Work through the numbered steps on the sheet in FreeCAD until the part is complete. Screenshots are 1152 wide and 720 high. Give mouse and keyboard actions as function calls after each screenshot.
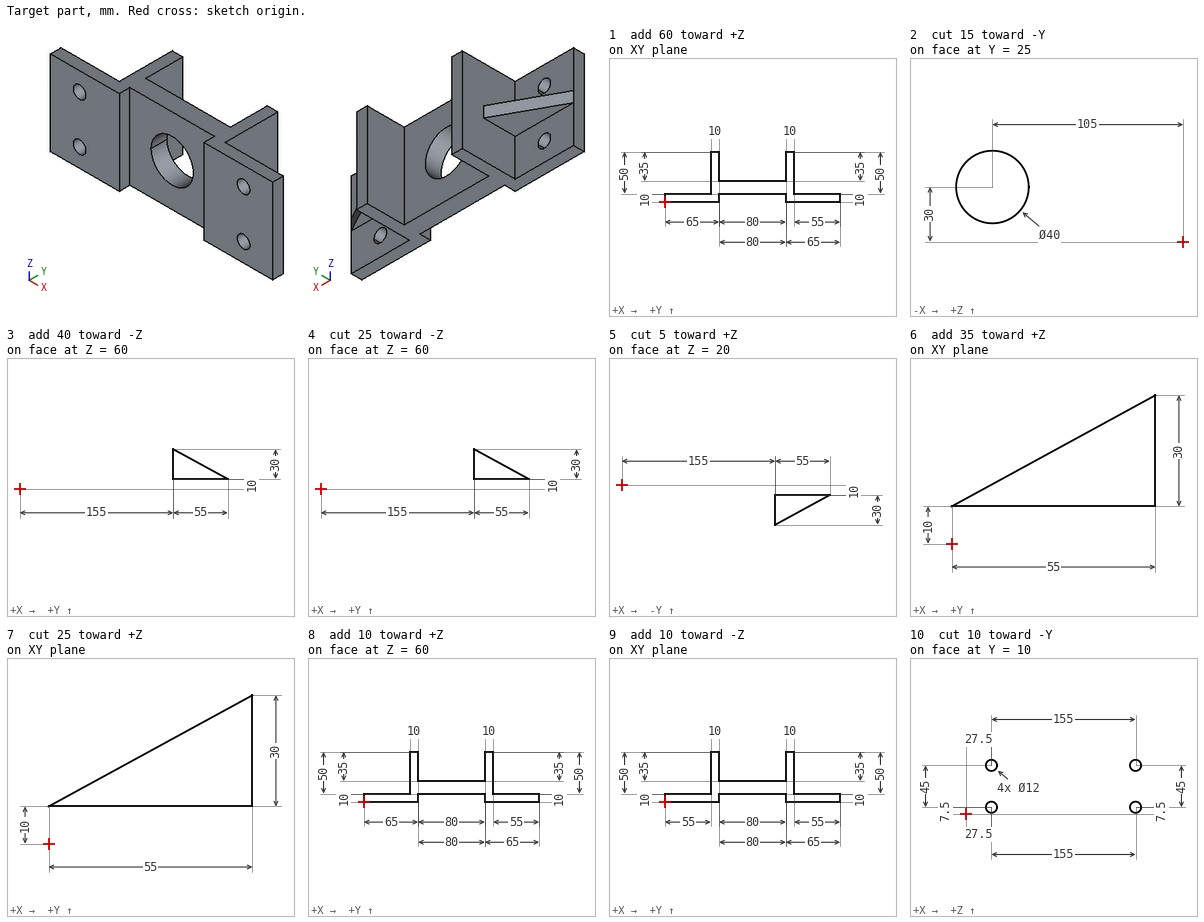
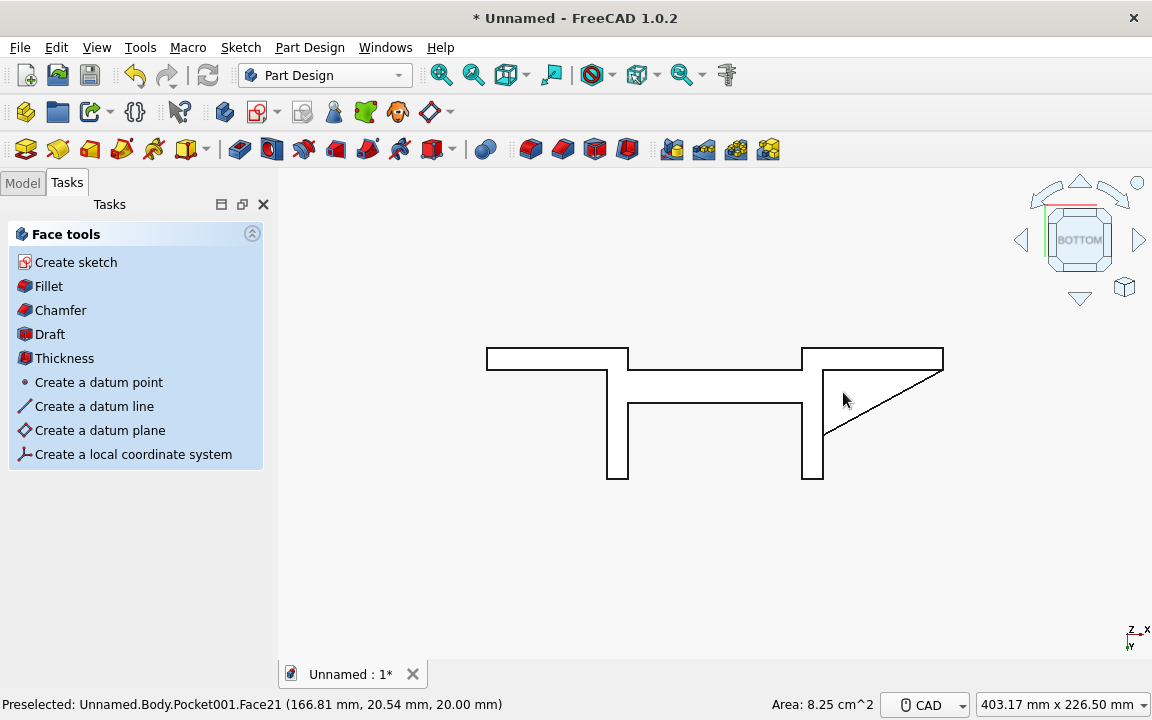
click(258, 112)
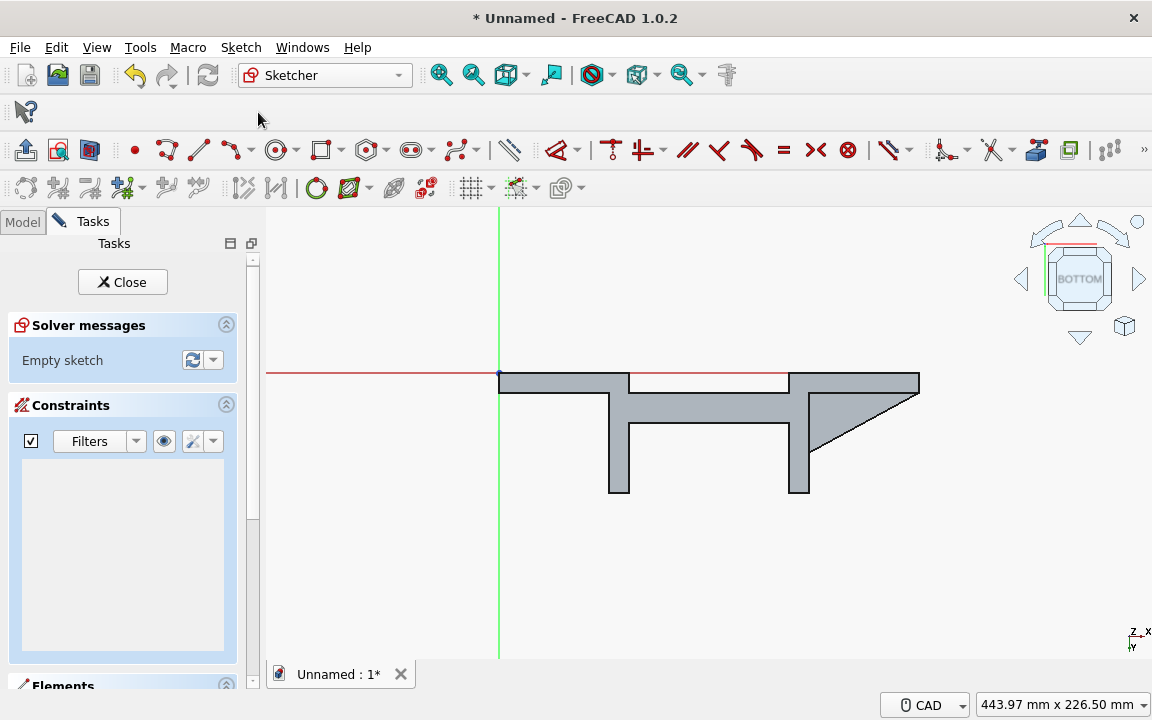
key(q)
key(s)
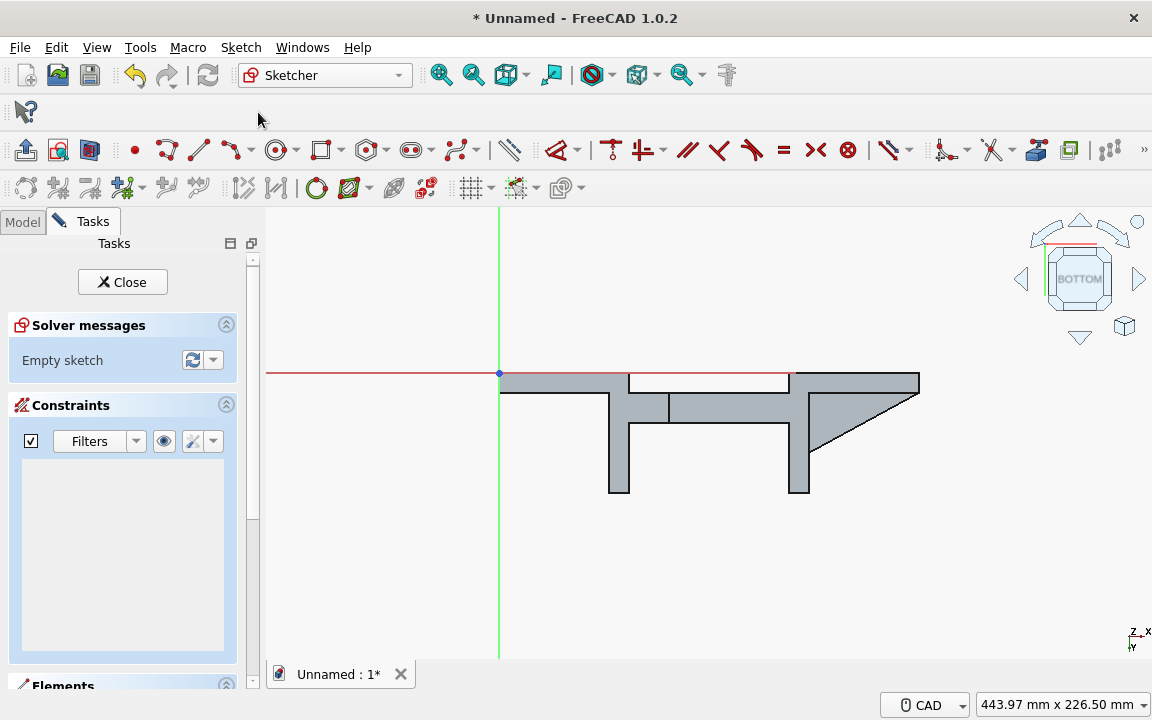
scroll(937, 420, up, 7)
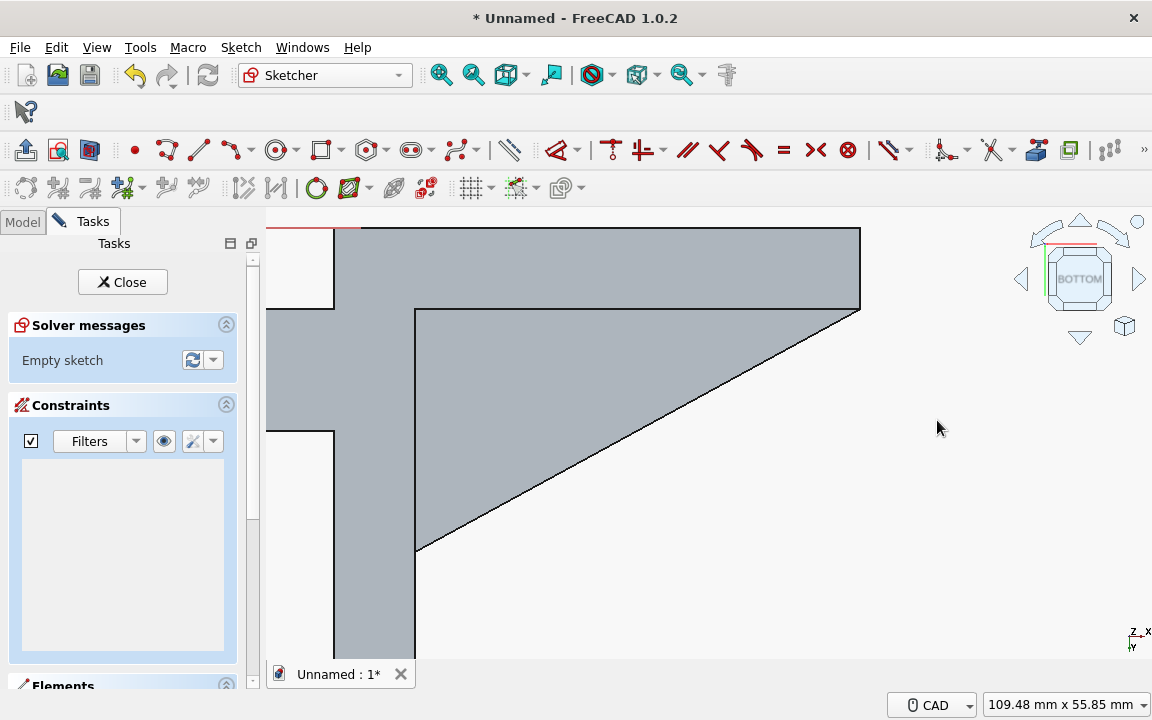
key(g)
key(m)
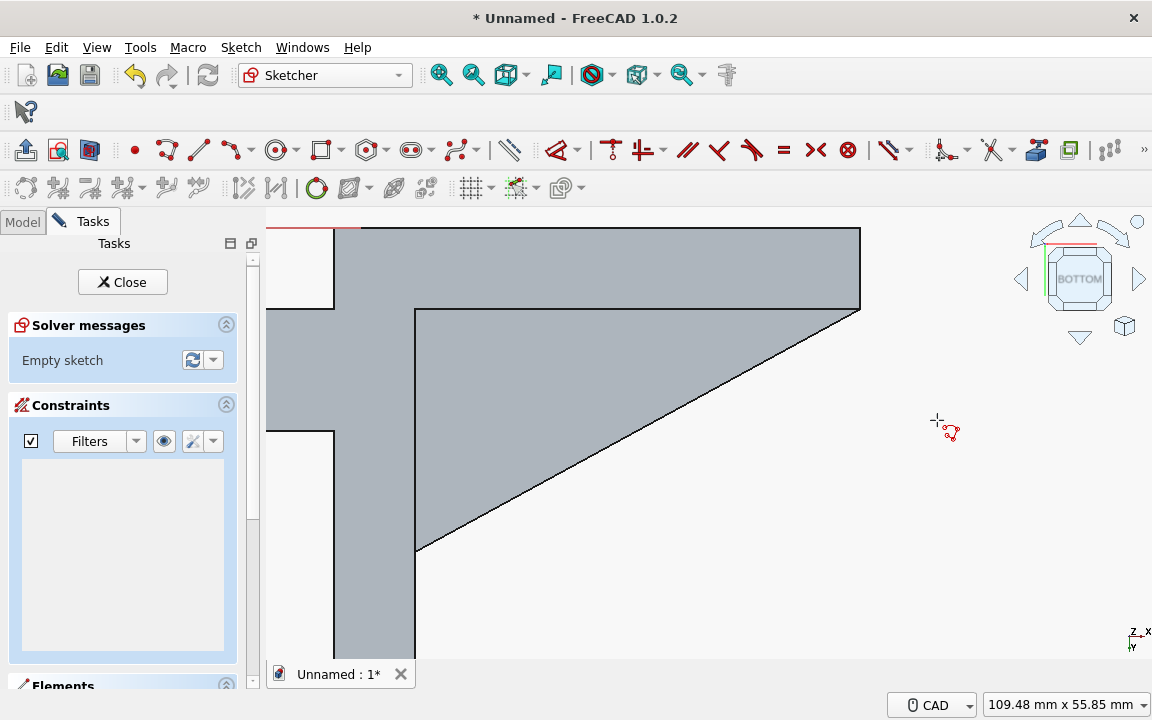
click(415, 309)
click(415, 552)
click(860, 309)
click(415, 310)
key(Escape)
key(Escape)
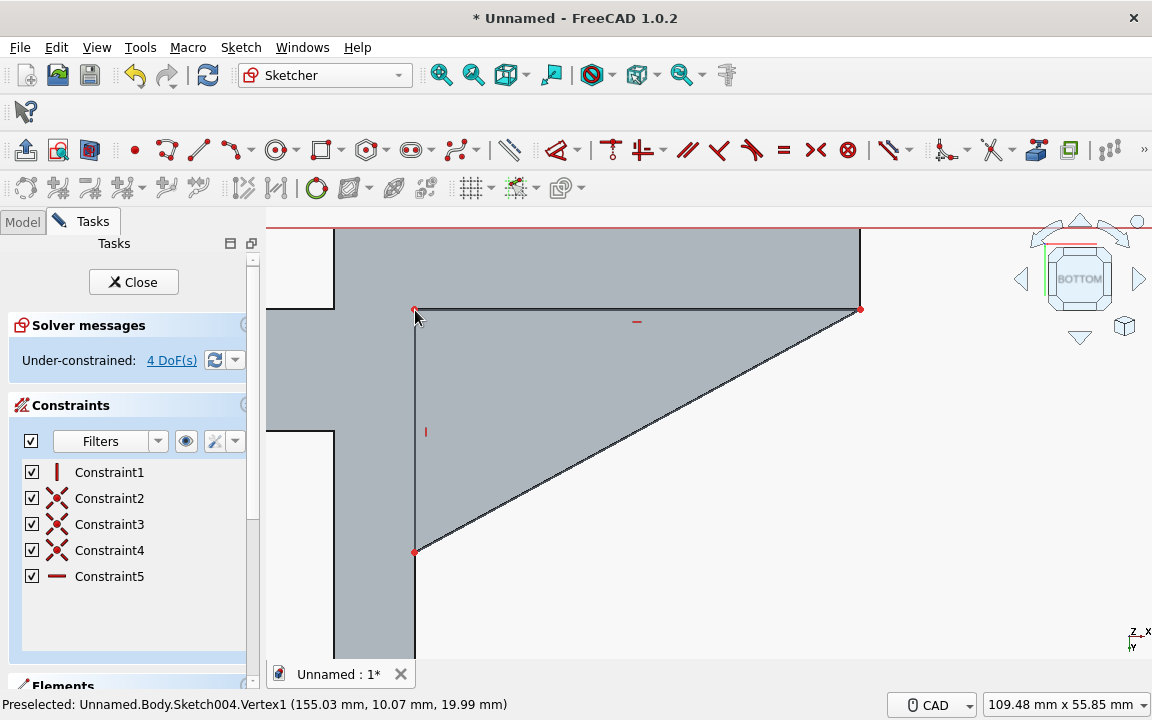
click(556, 150)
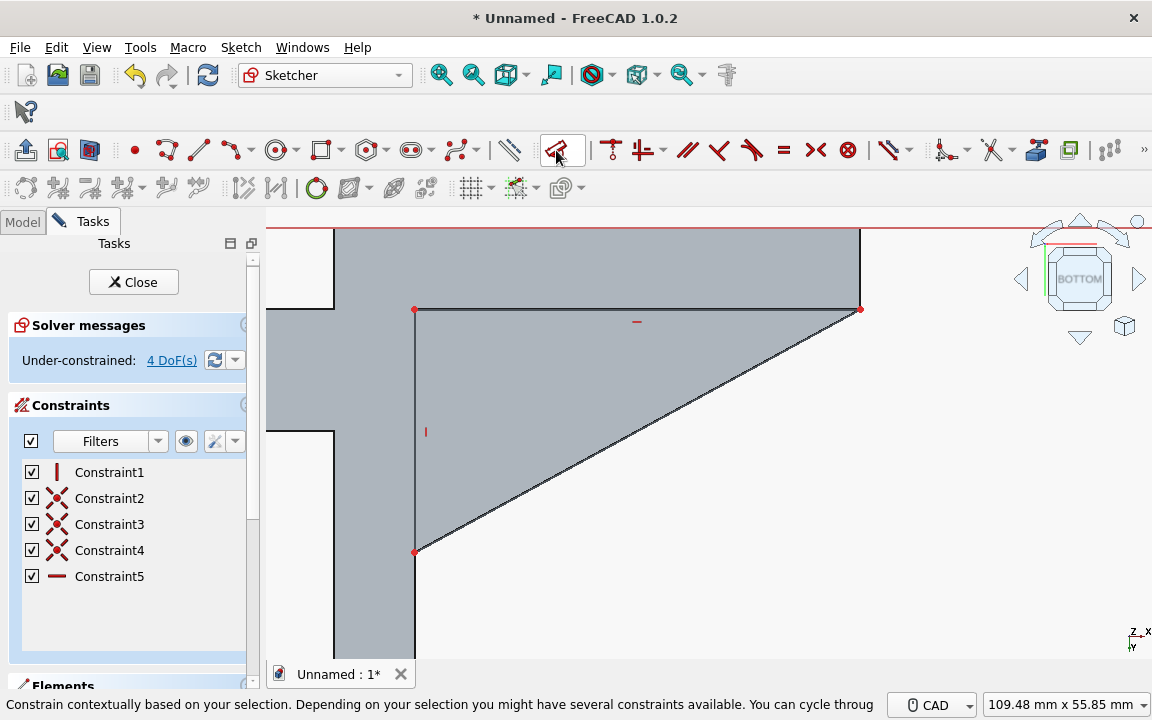
click(415, 383)
click(381, 432)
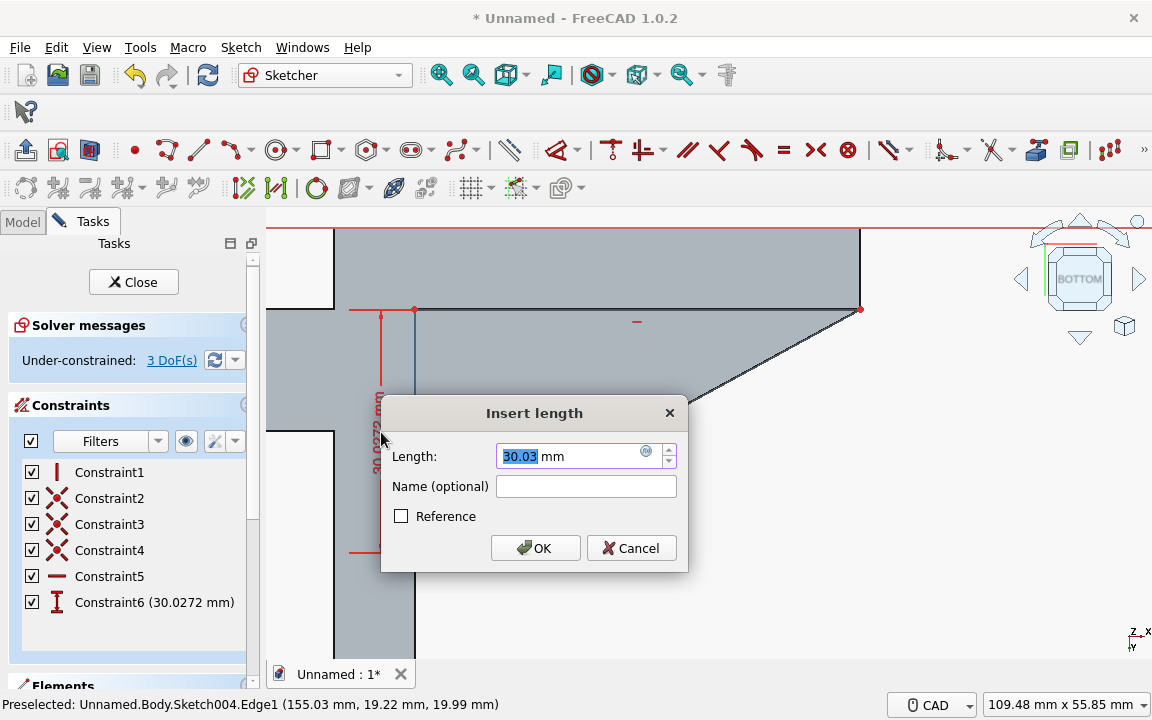
text(30)
key(Return)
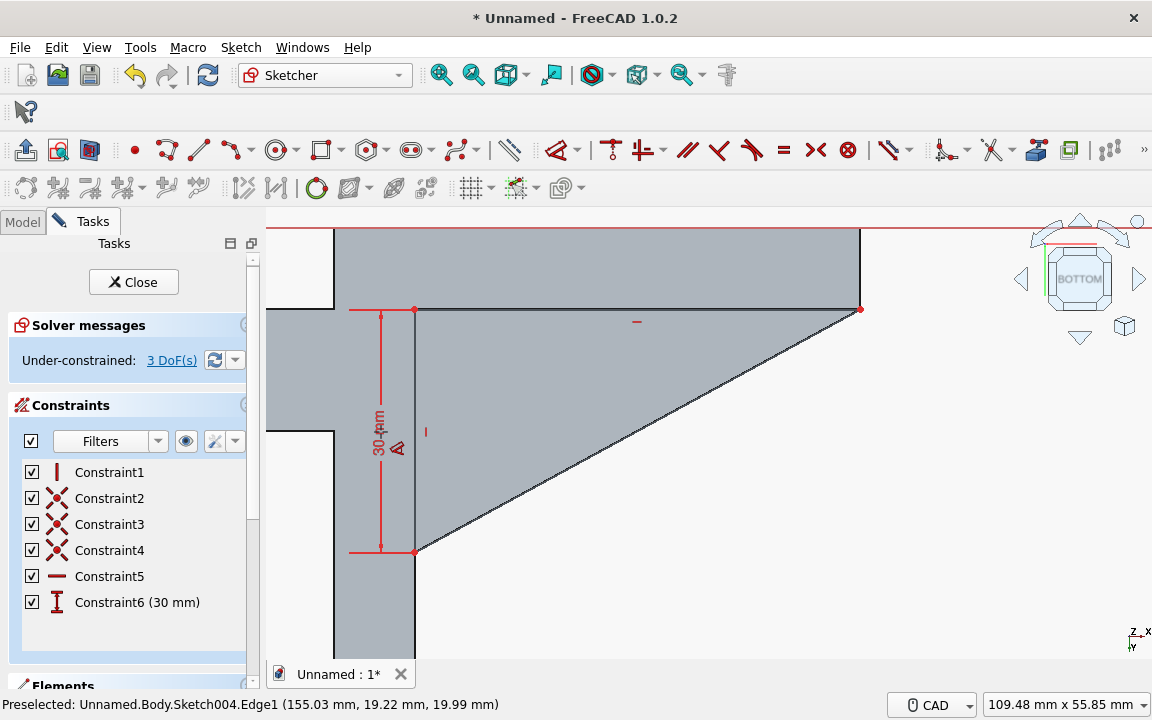
click(726, 310)
click(637, 276)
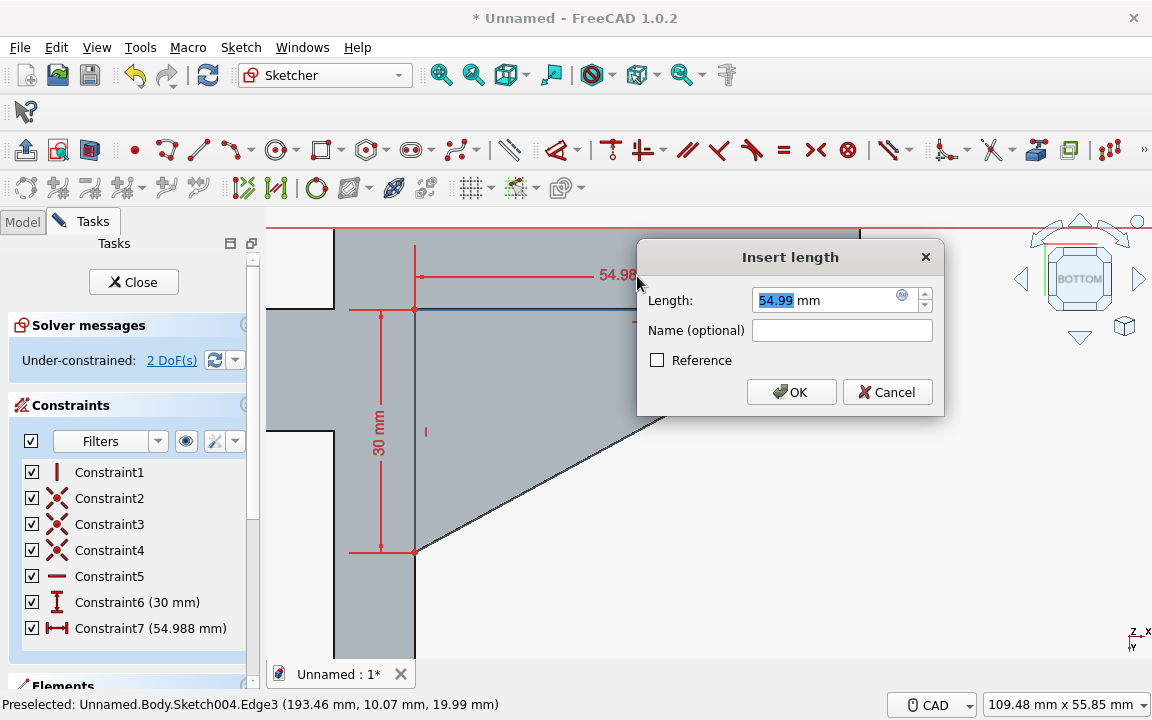
text(55)
key(Return)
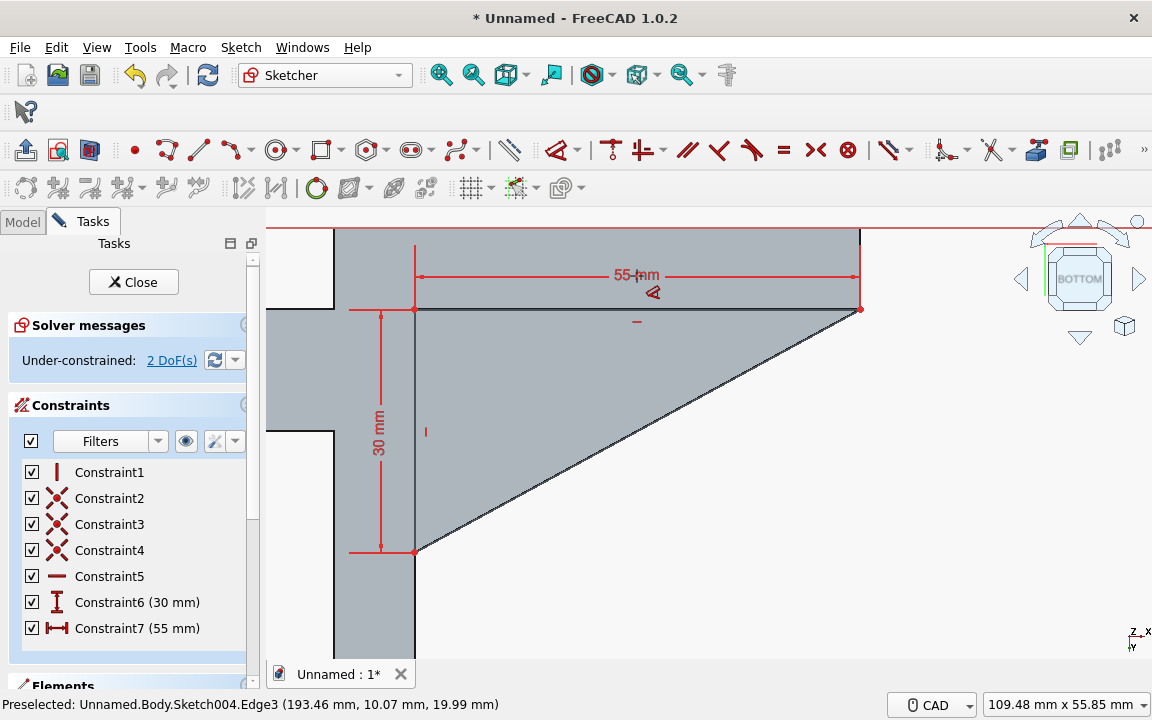
click(415, 310)
click(449, 273)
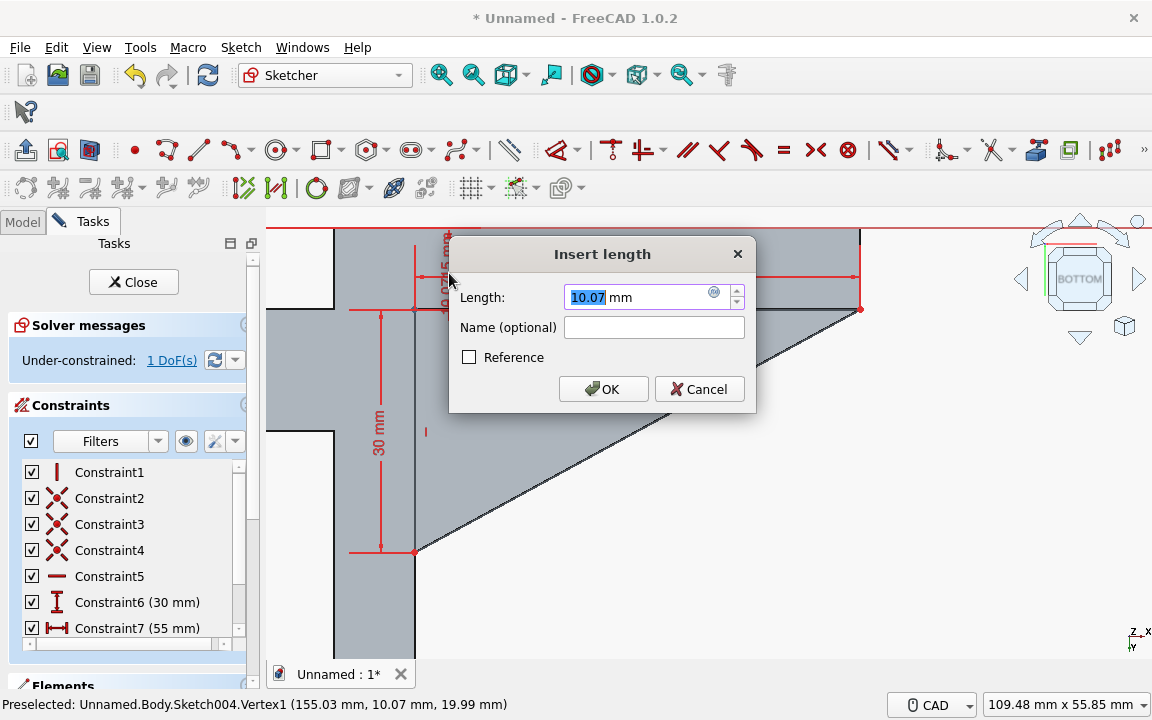
text(10)
key(Return)